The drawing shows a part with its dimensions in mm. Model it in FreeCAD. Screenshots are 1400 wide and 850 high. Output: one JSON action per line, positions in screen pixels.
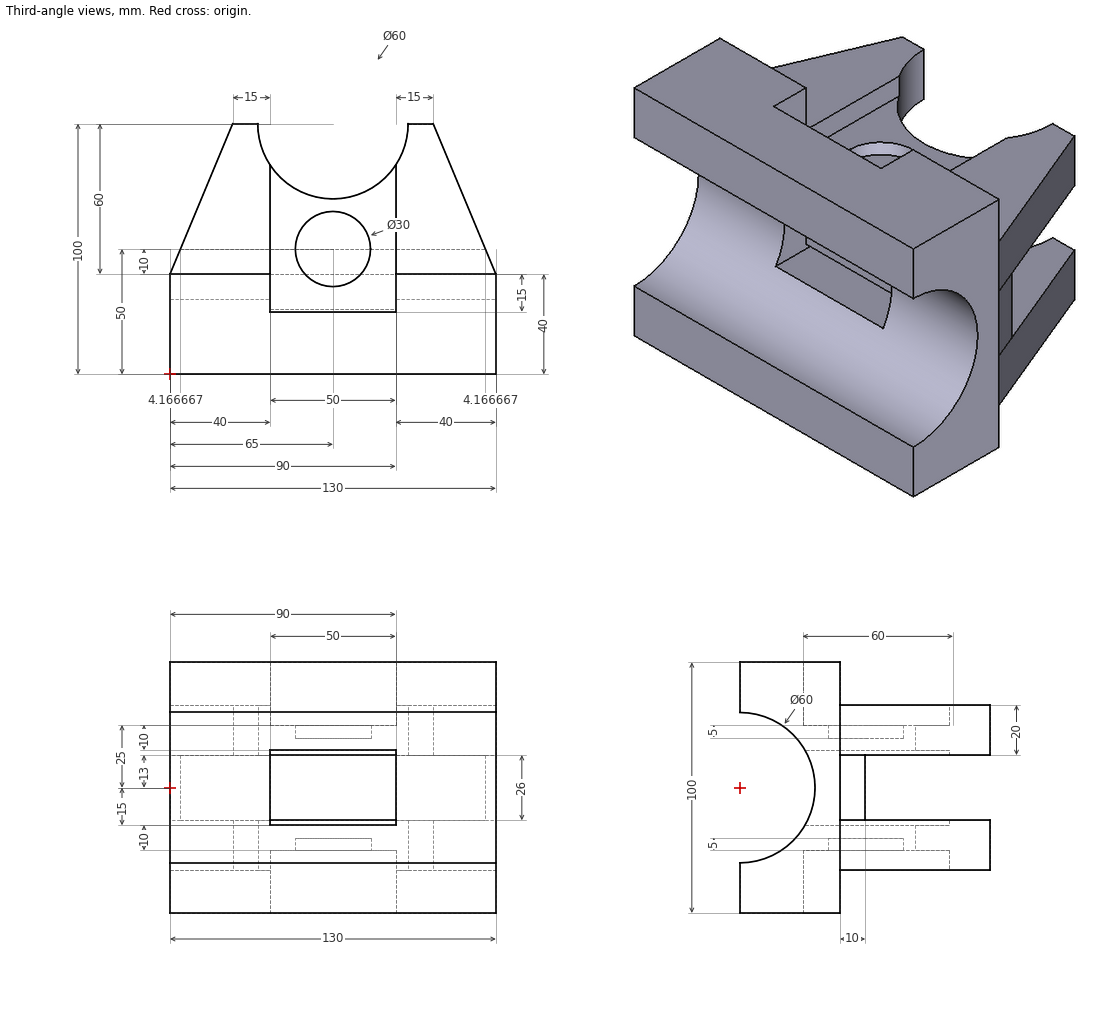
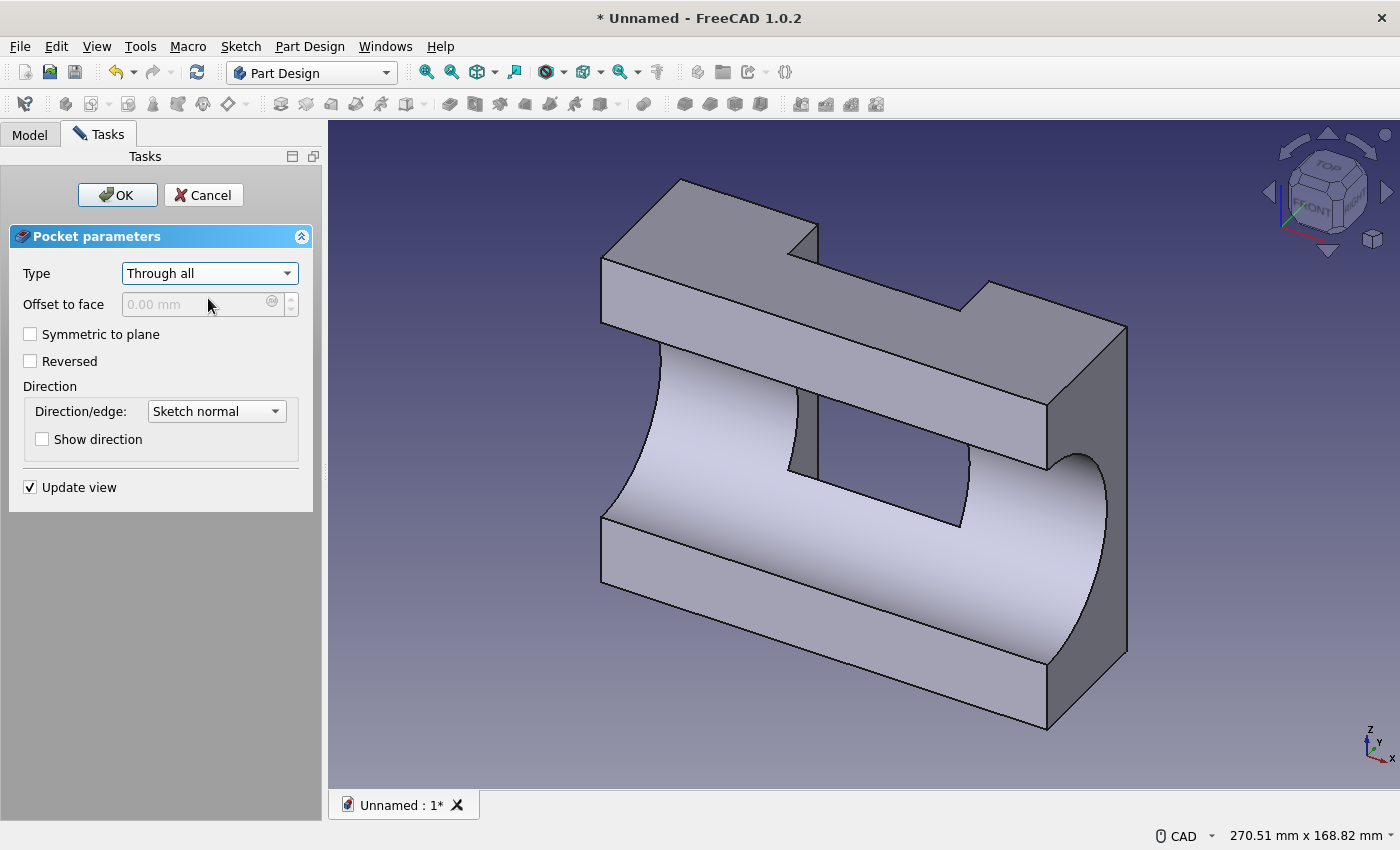
{"action": "left_click", "coordinate": [118, 195]}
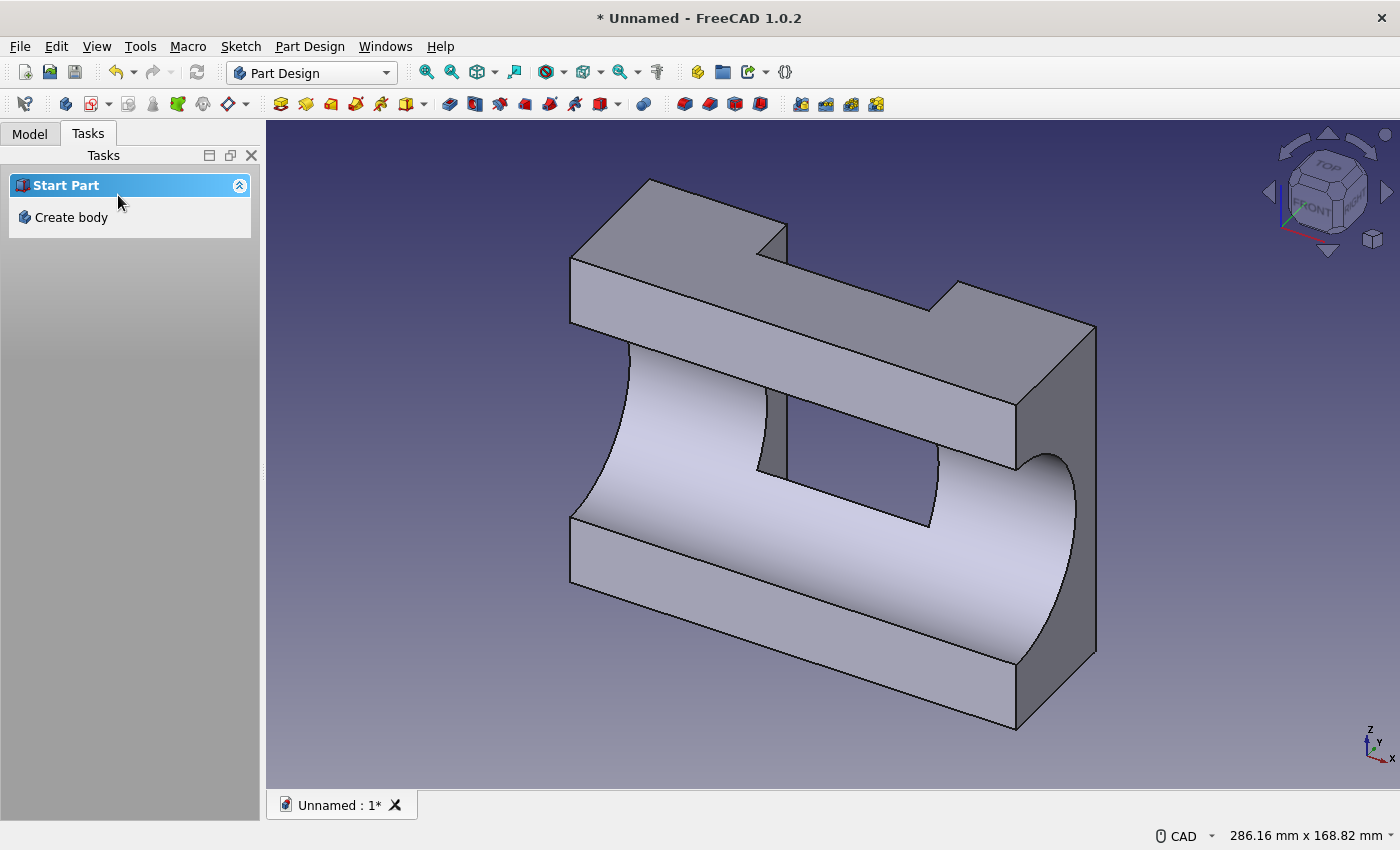
{"action": "key", "text": "4"}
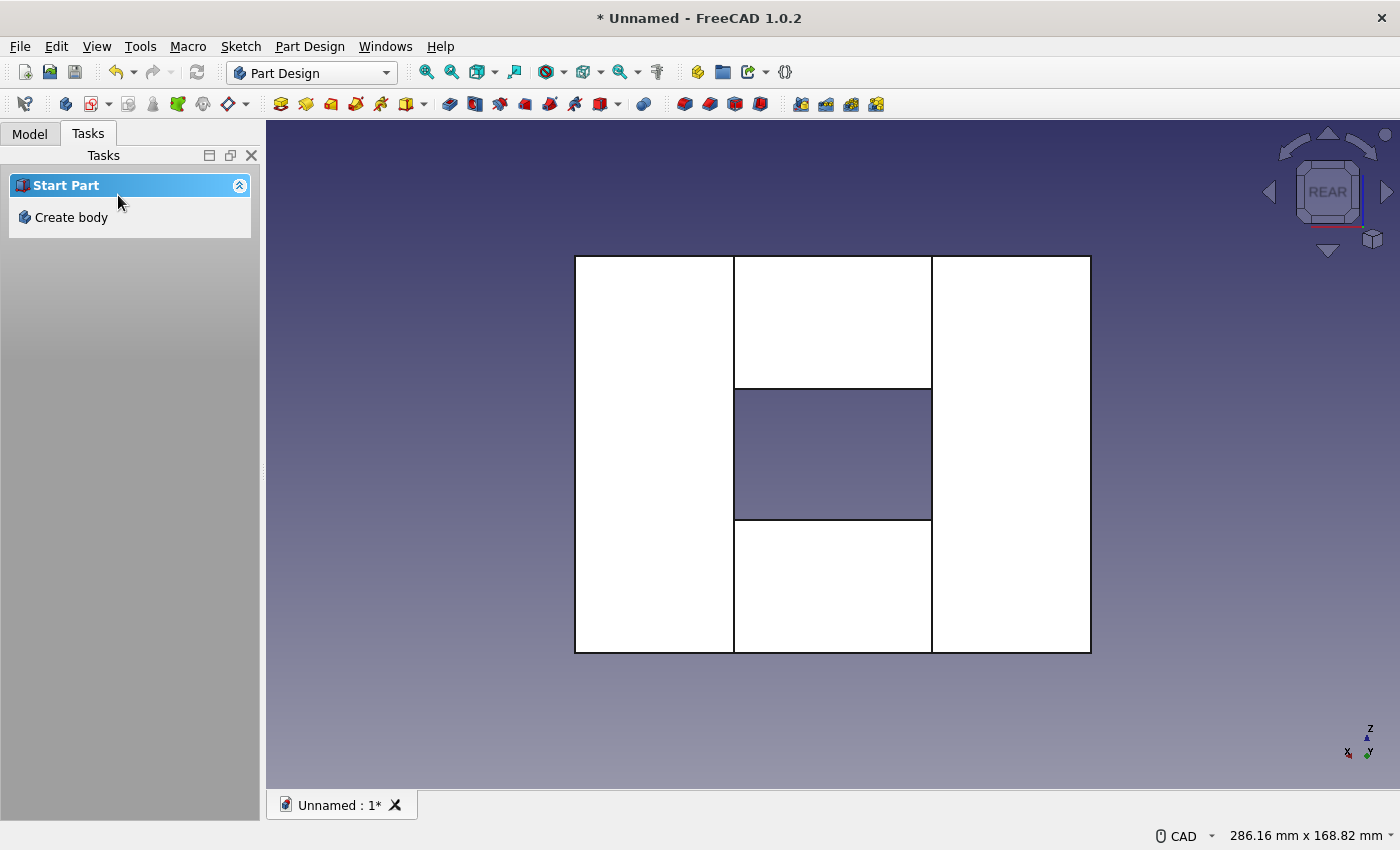
{"action": "left_click", "coordinate": [805, 585]}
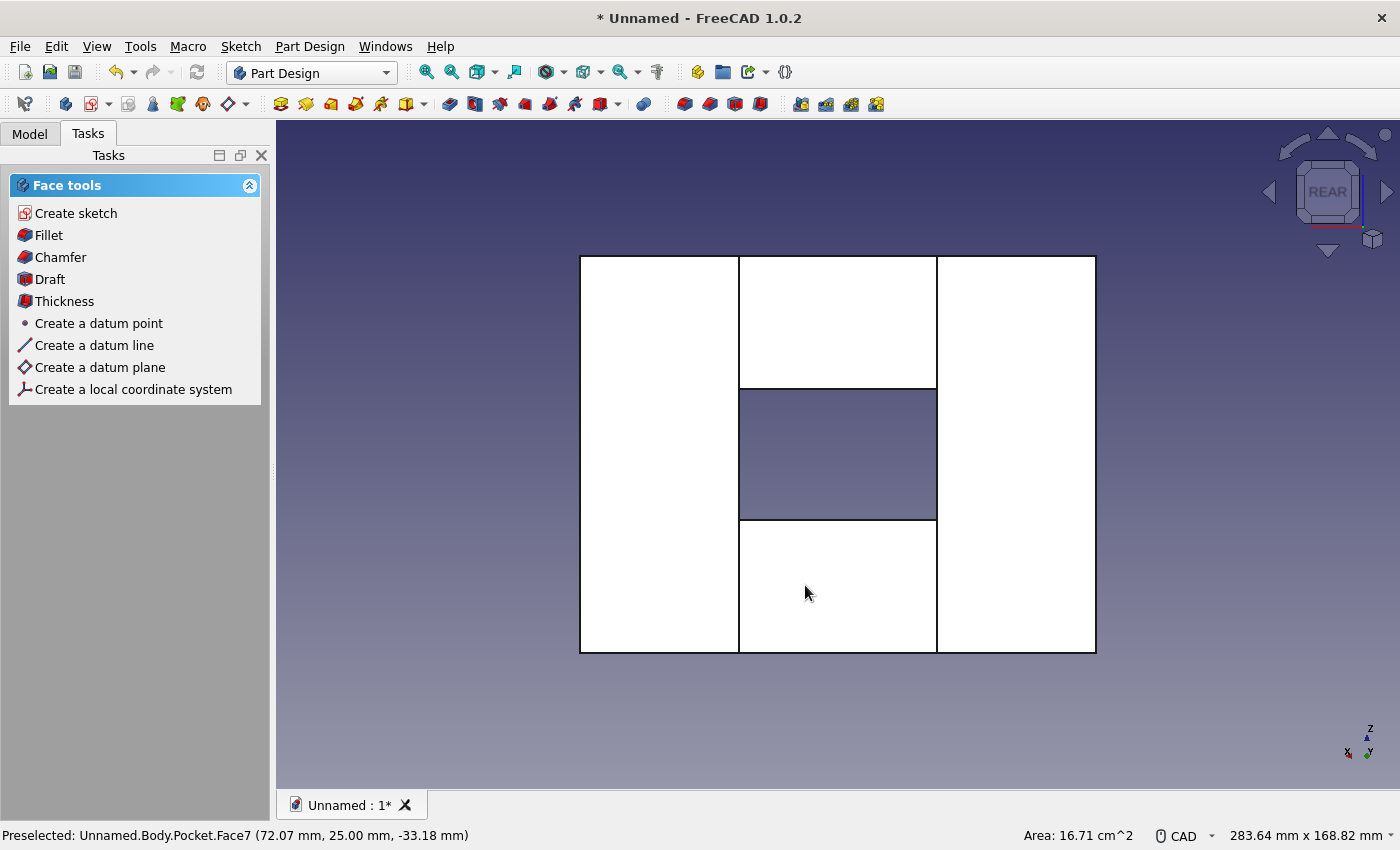
{"action": "left_click", "coordinate": [90, 104]}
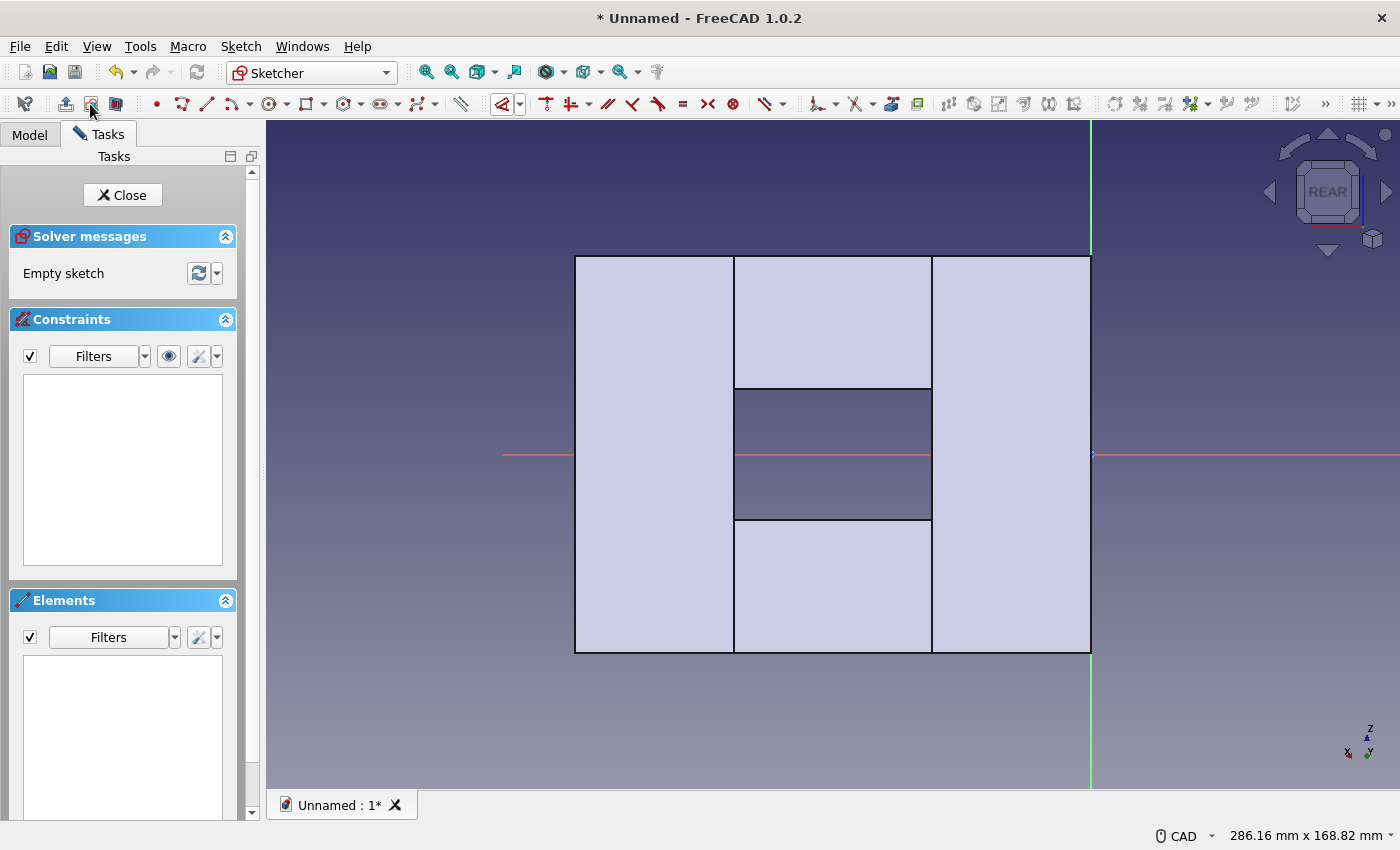
{"action": "scroll", "coordinate": [1092, 345], "scroll_direction": "up", "scroll_amount": 3}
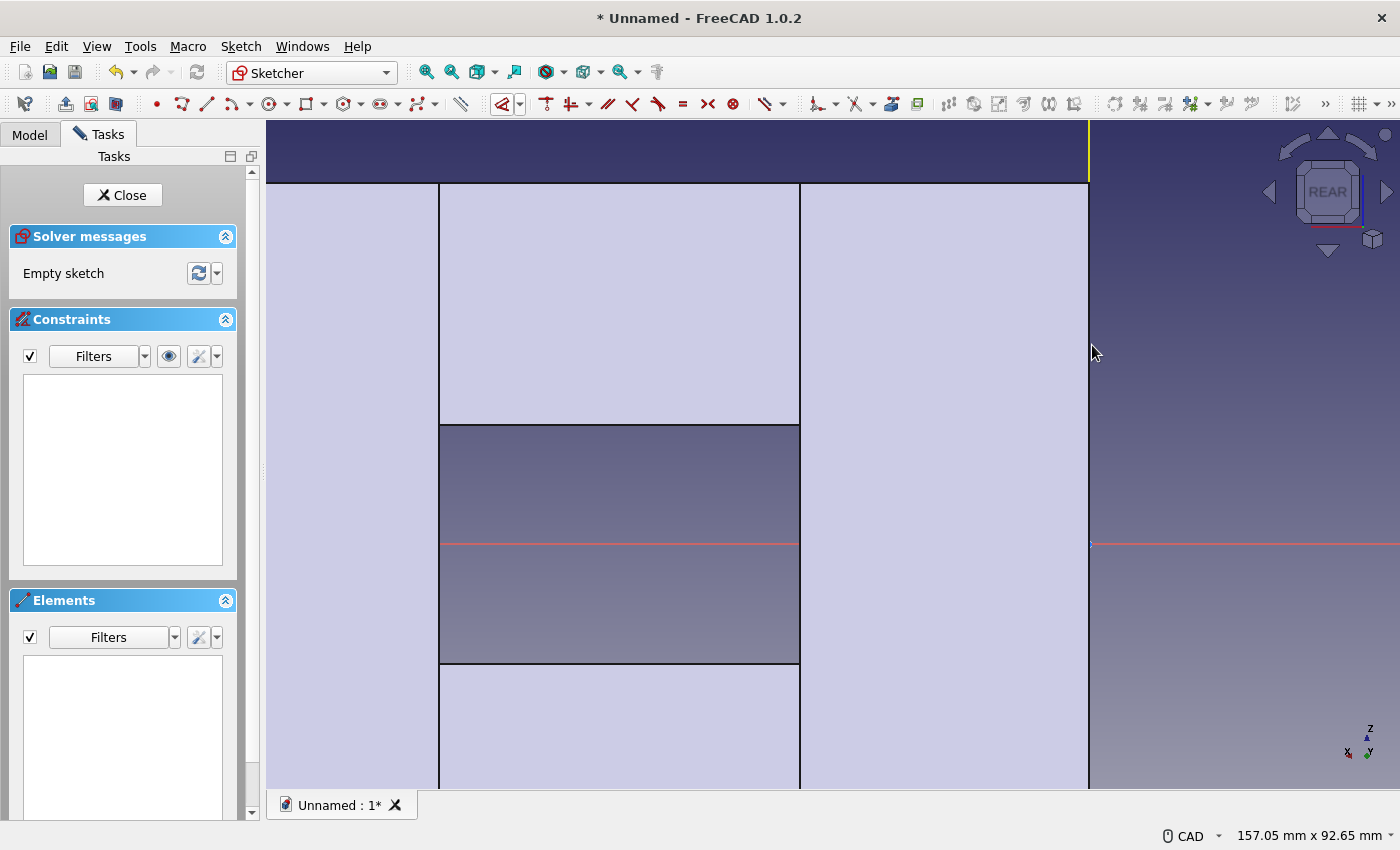
{"action": "left_click", "coordinate": [306, 104]}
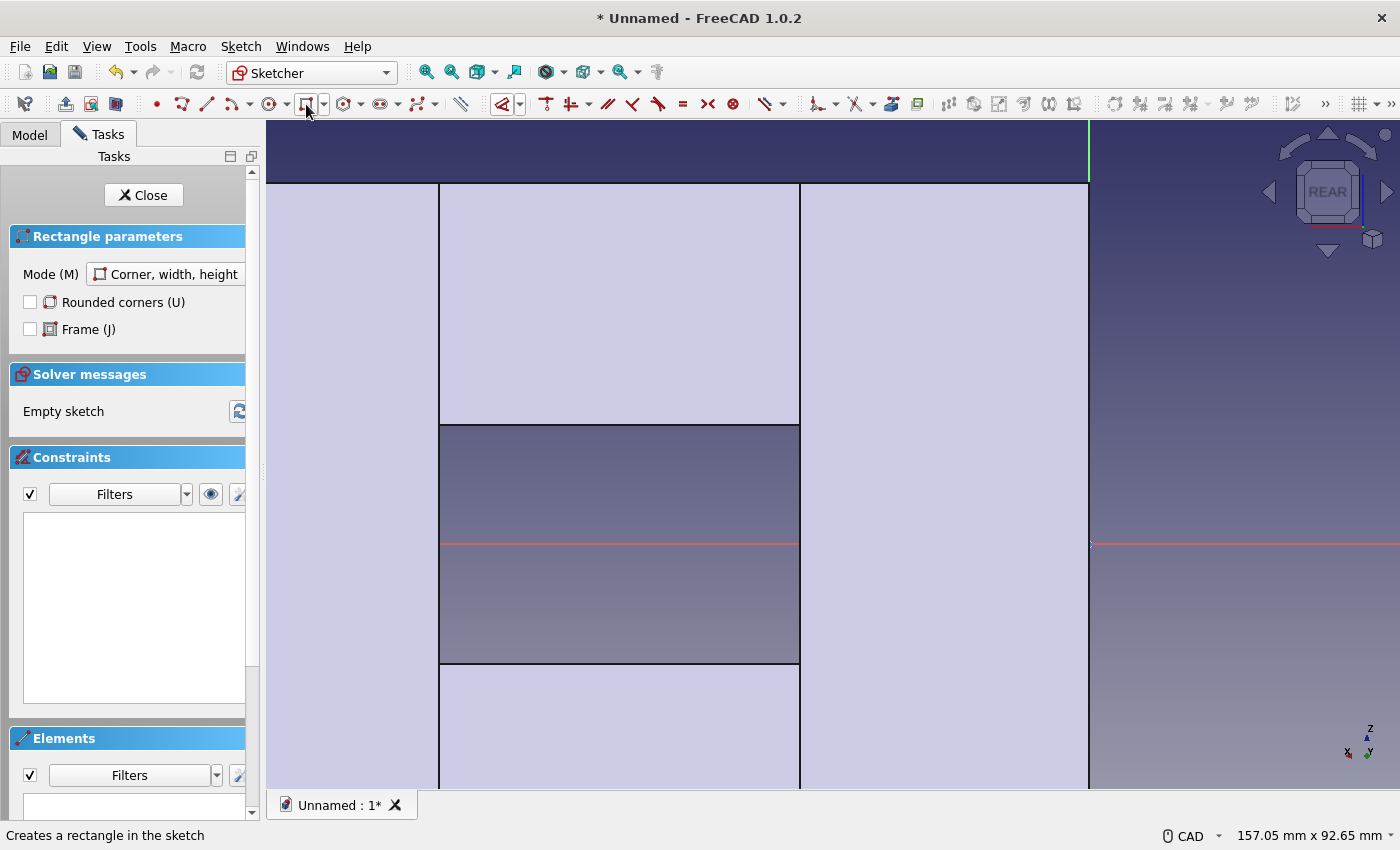
{"action": "left_click", "coordinate": [439, 364]}
{"action": "mouse_move", "coordinate": [800, 436]}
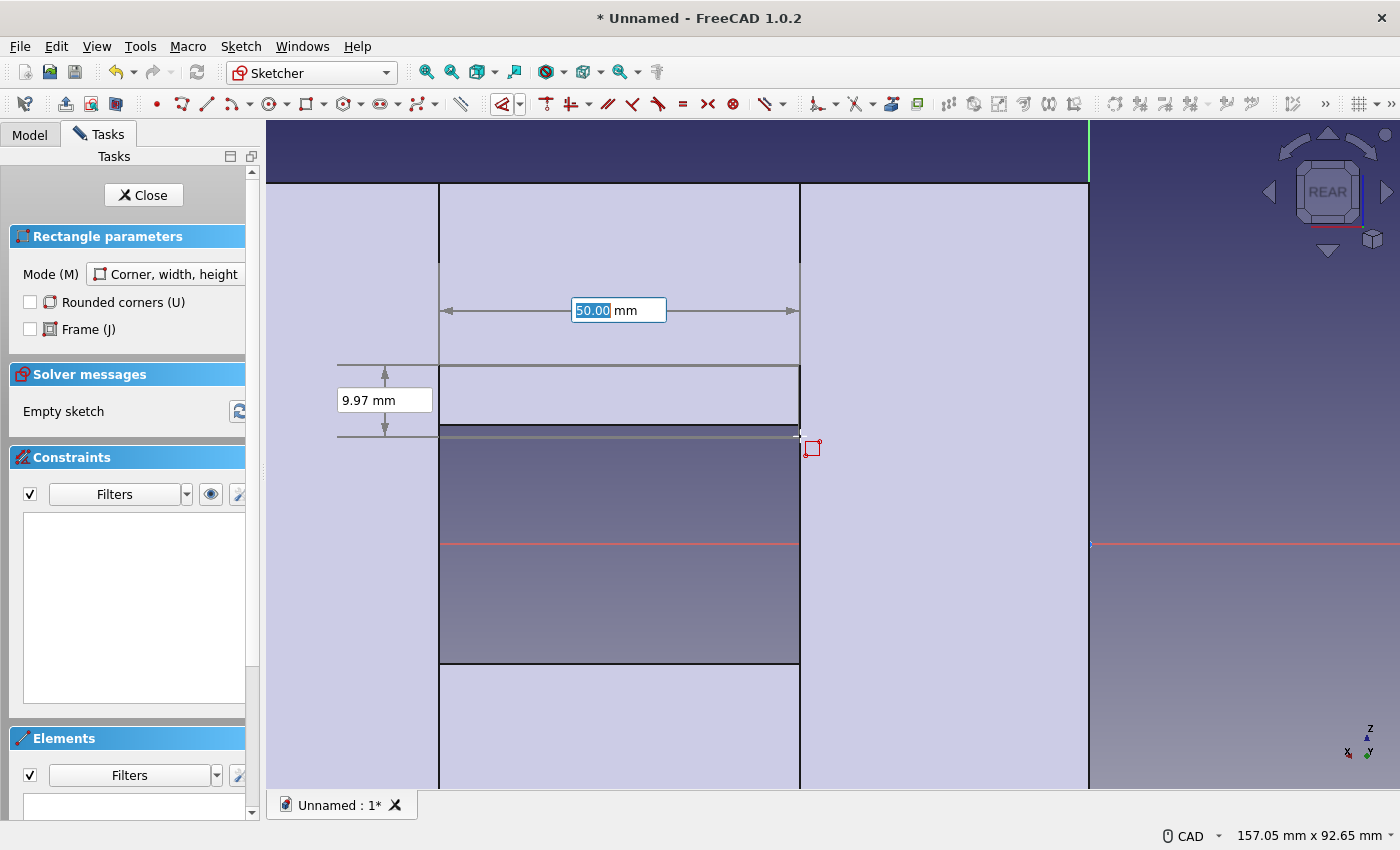
{"action": "type", "text": "50"}
{"action": "key", "text": "Tab"}
{"action": "type", "text": "10"}
{"action": "key", "text": "Return"}
{"action": "key", "text": "Escape"}